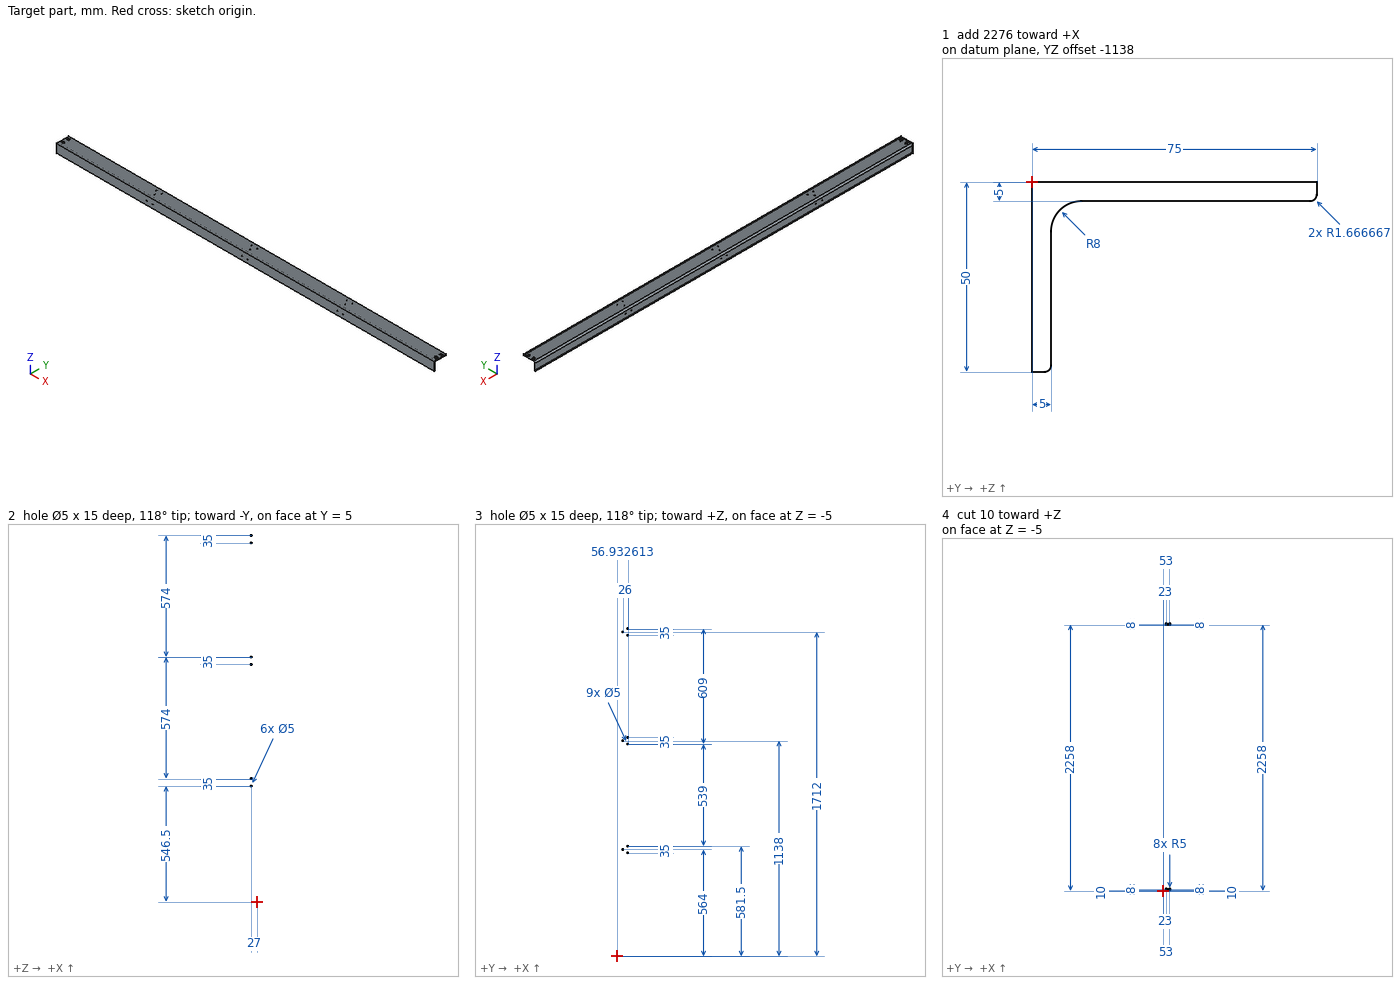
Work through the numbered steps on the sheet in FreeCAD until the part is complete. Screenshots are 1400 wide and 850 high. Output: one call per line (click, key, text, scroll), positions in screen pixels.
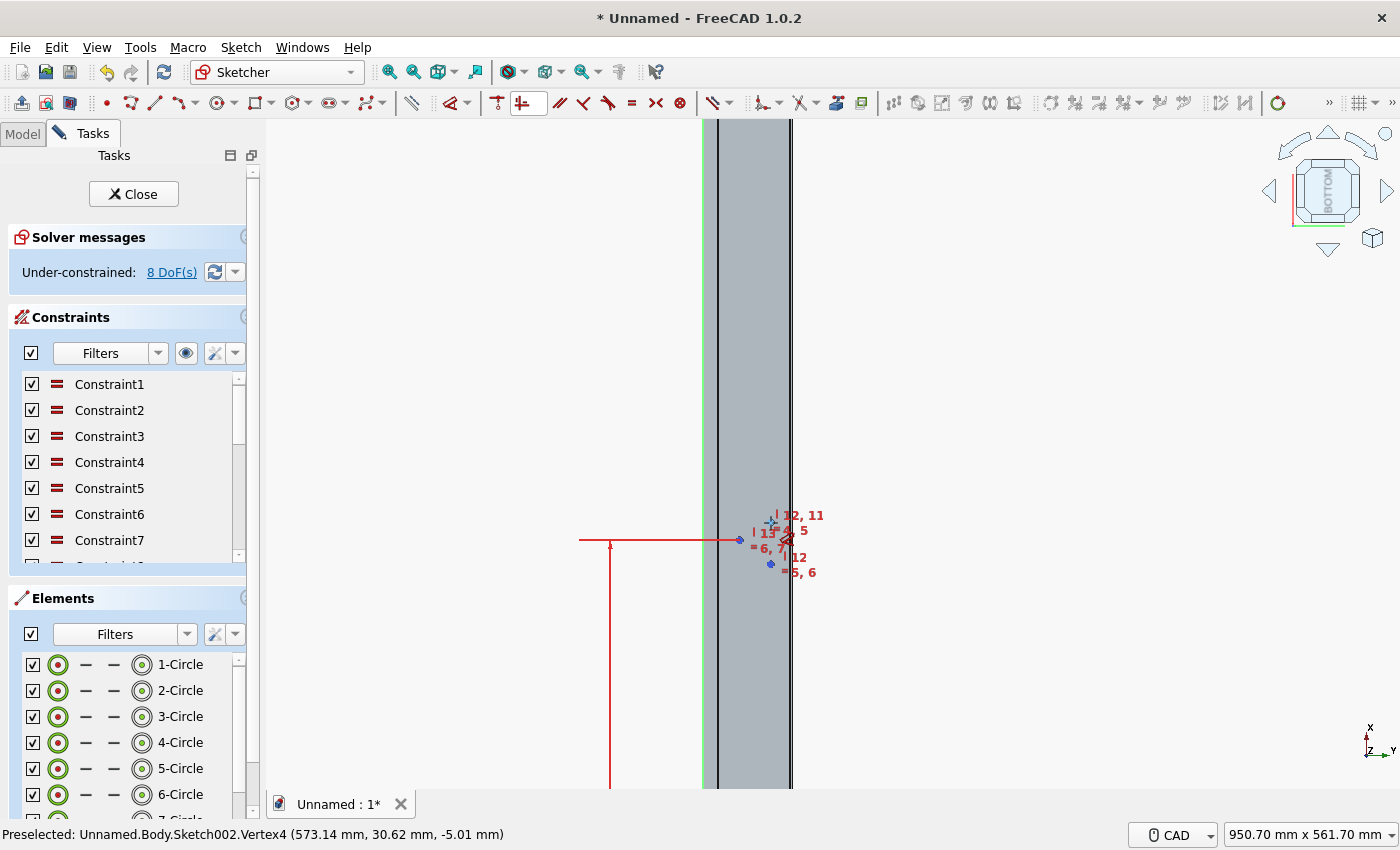
click(771, 522)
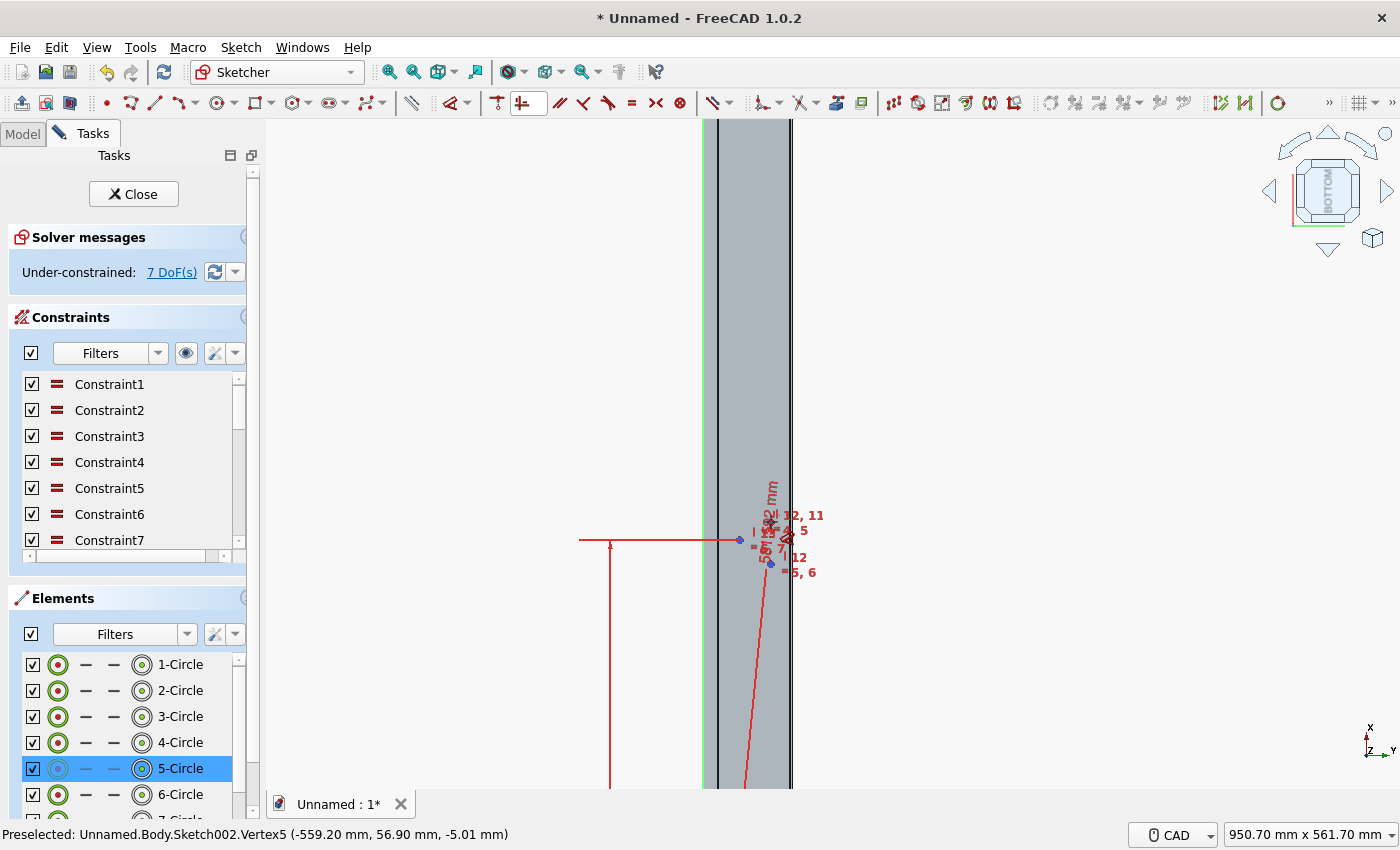
click(771, 564)
click(805, 543)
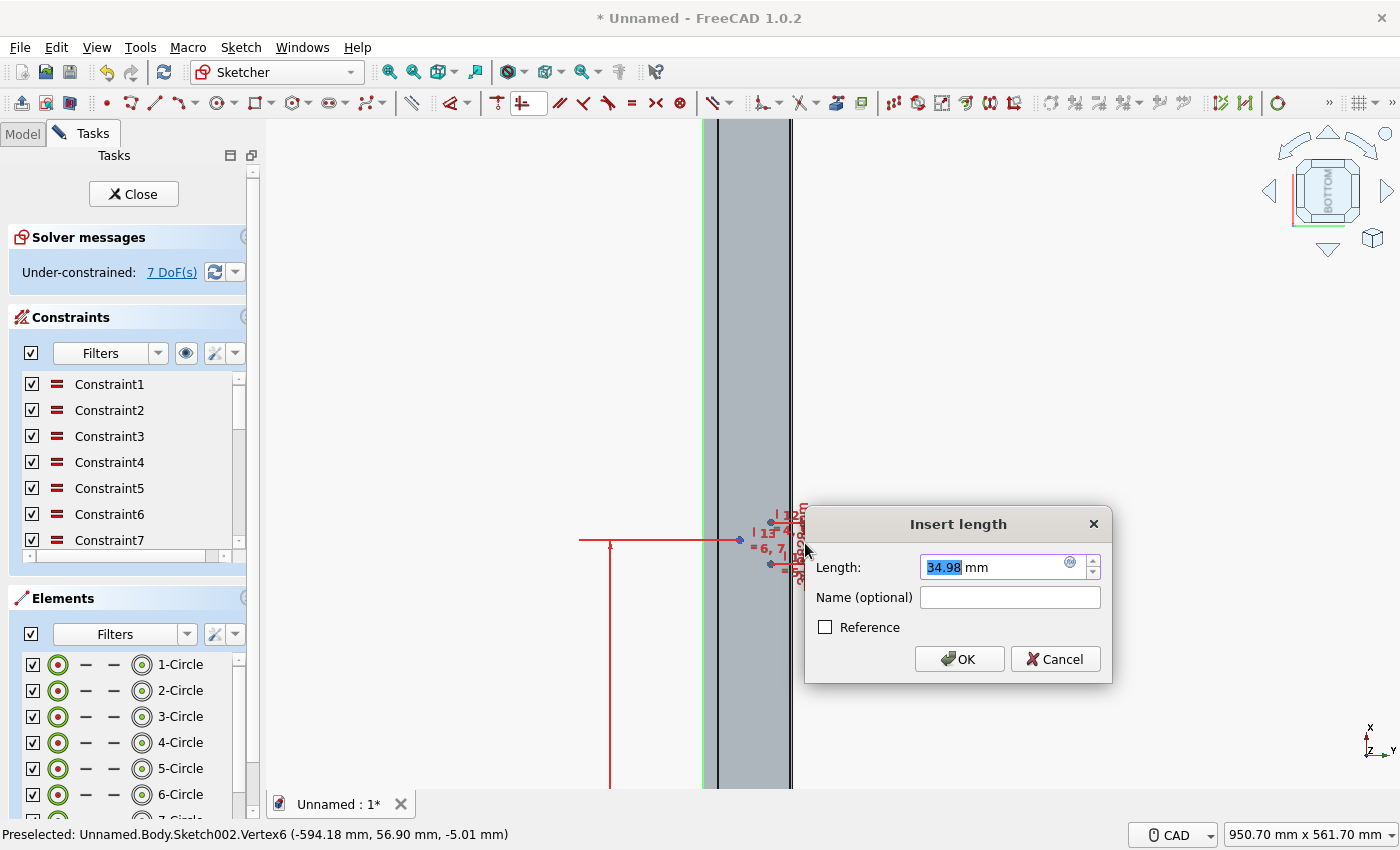
text(35)
key(Return)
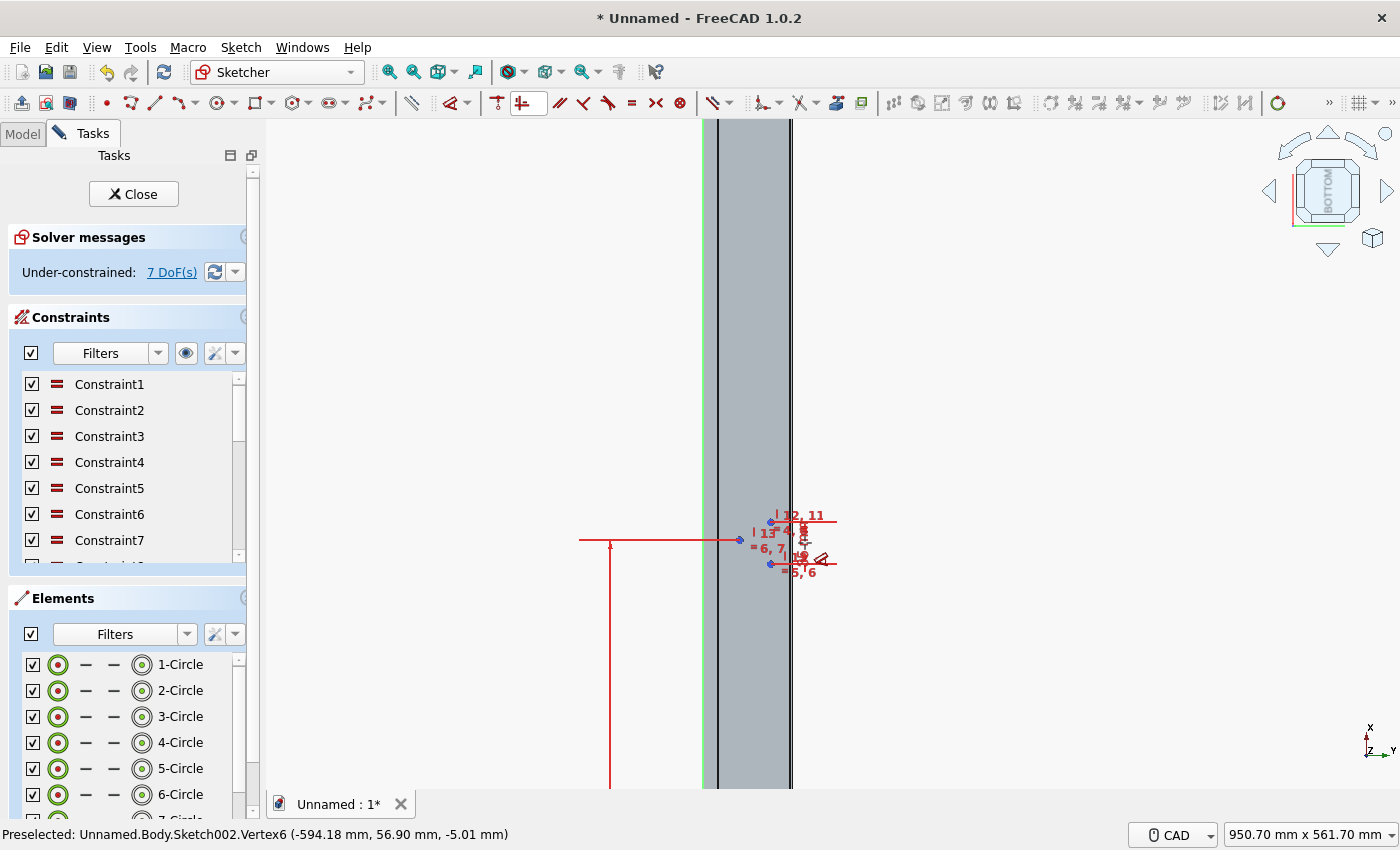
scroll(771, 523, down, 8)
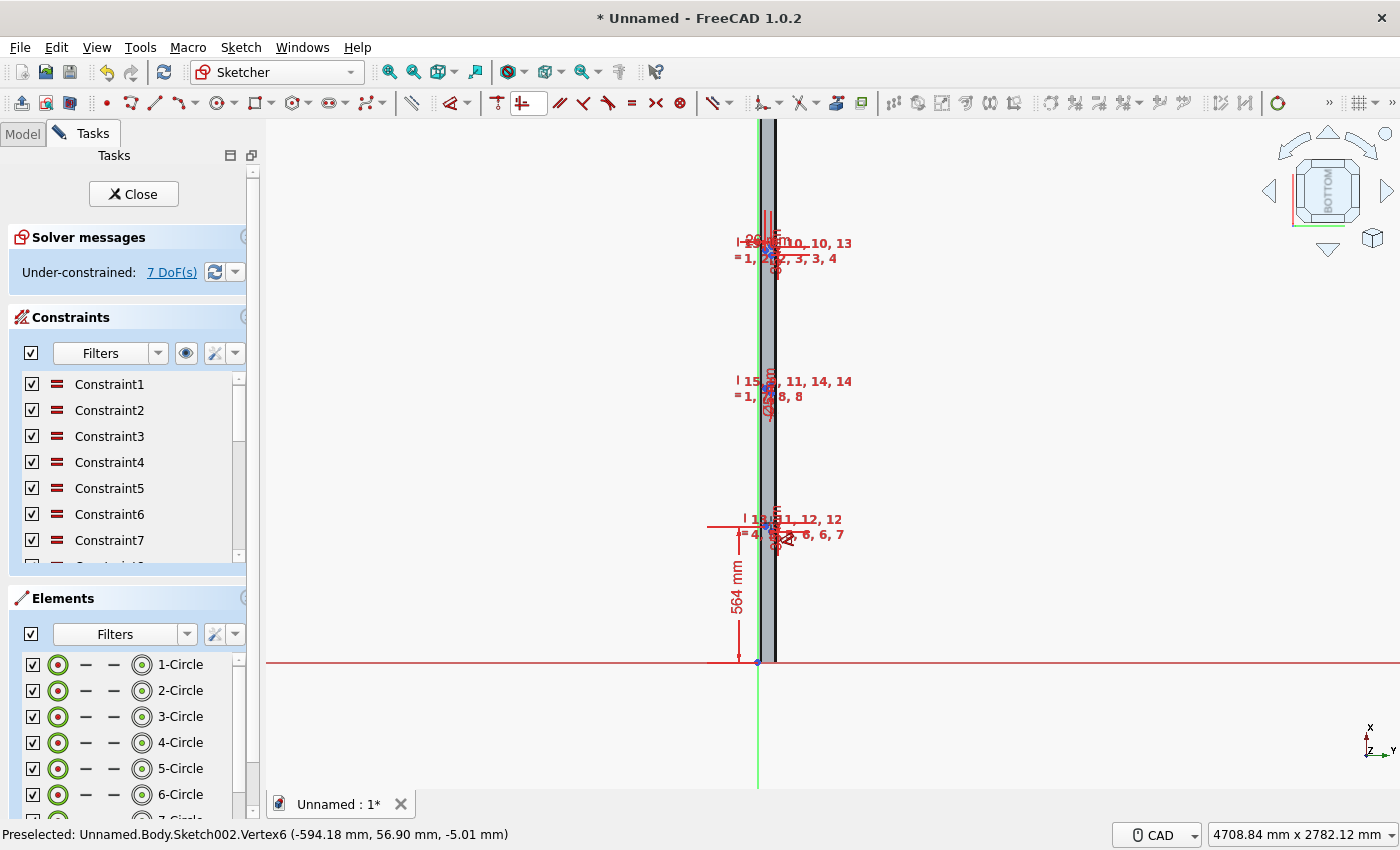
scroll(771, 394, up, 8)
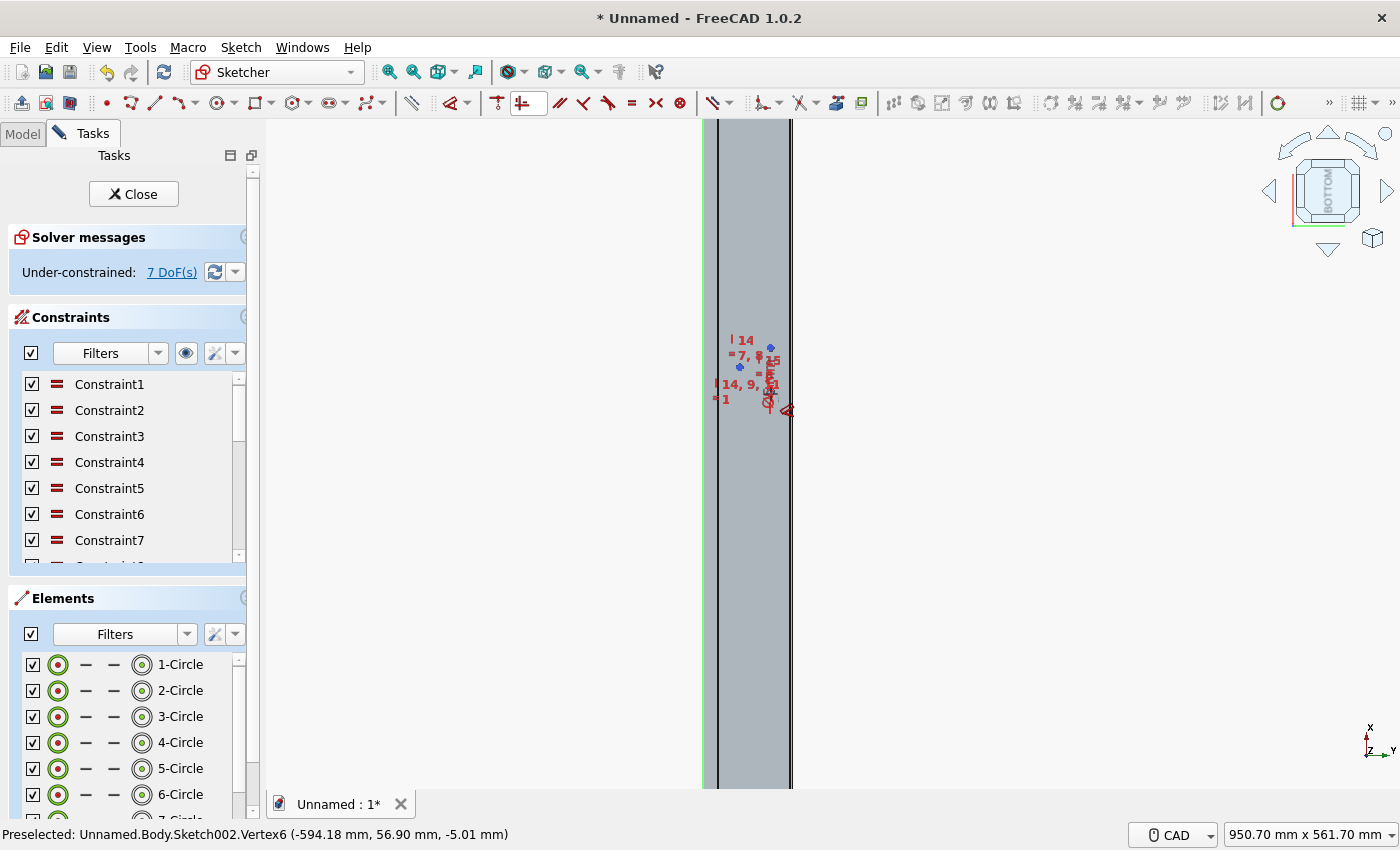
click(771, 391)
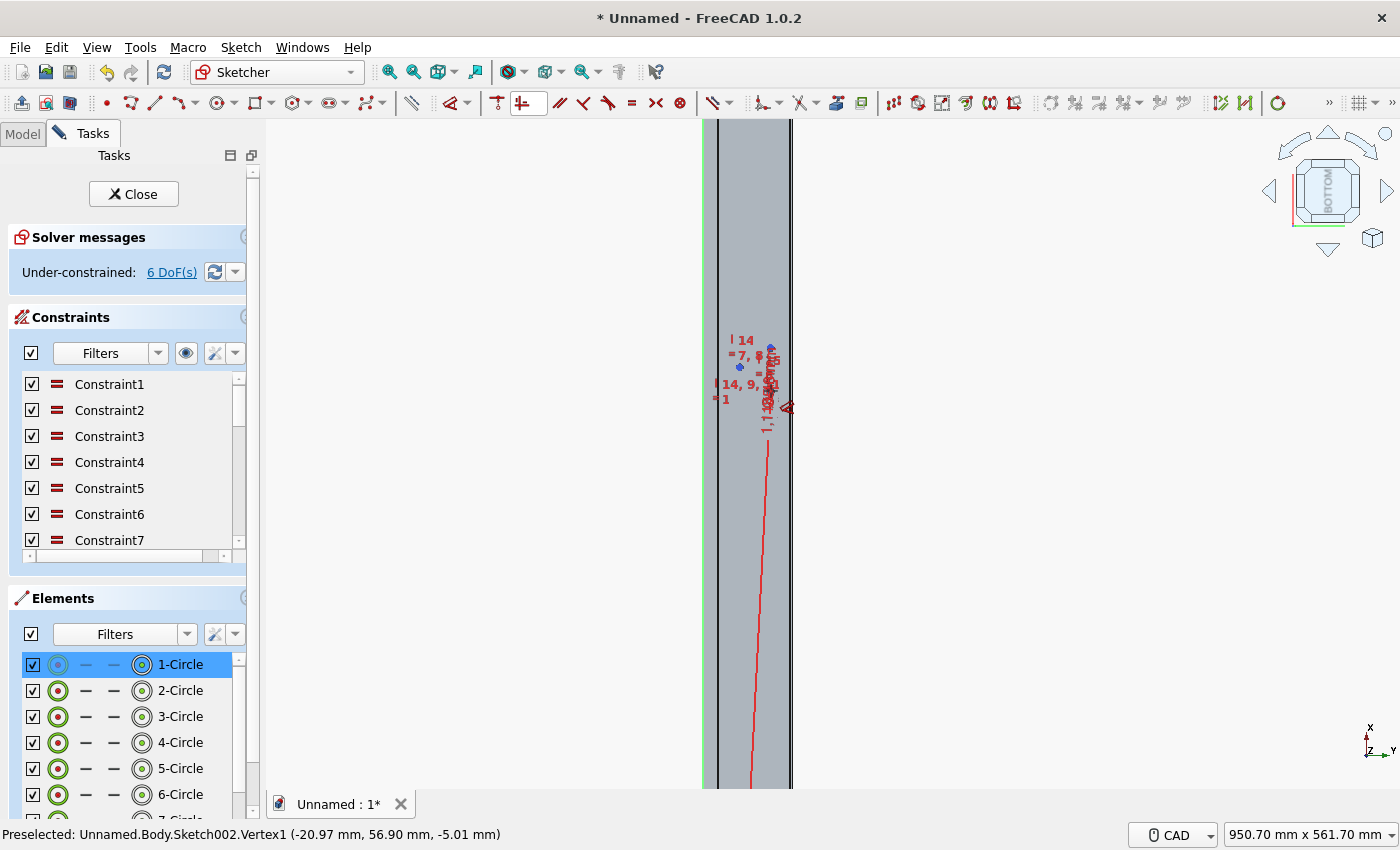
click(771, 348)
click(805, 360)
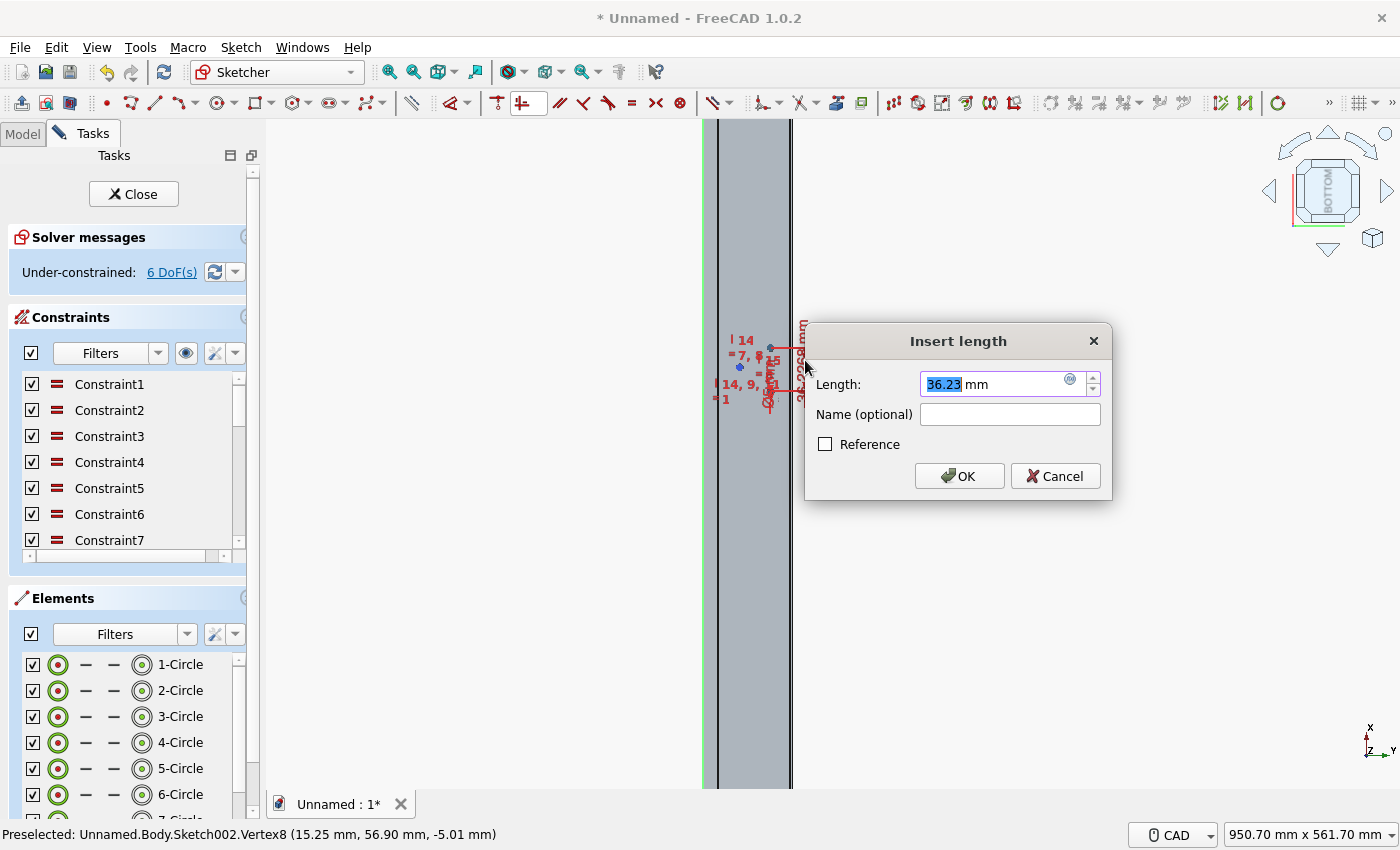
text(35)
key(Return)